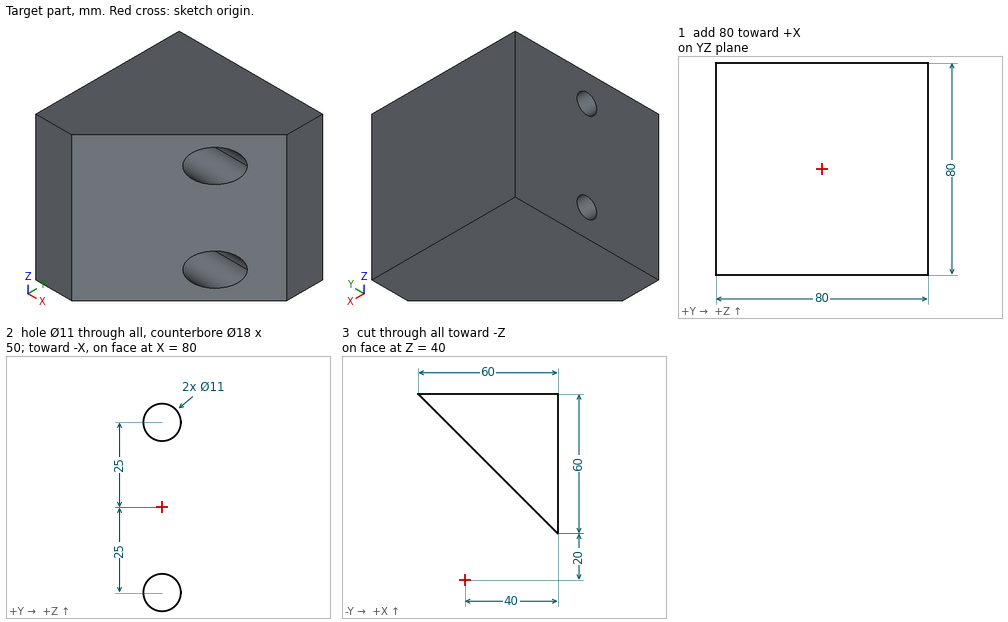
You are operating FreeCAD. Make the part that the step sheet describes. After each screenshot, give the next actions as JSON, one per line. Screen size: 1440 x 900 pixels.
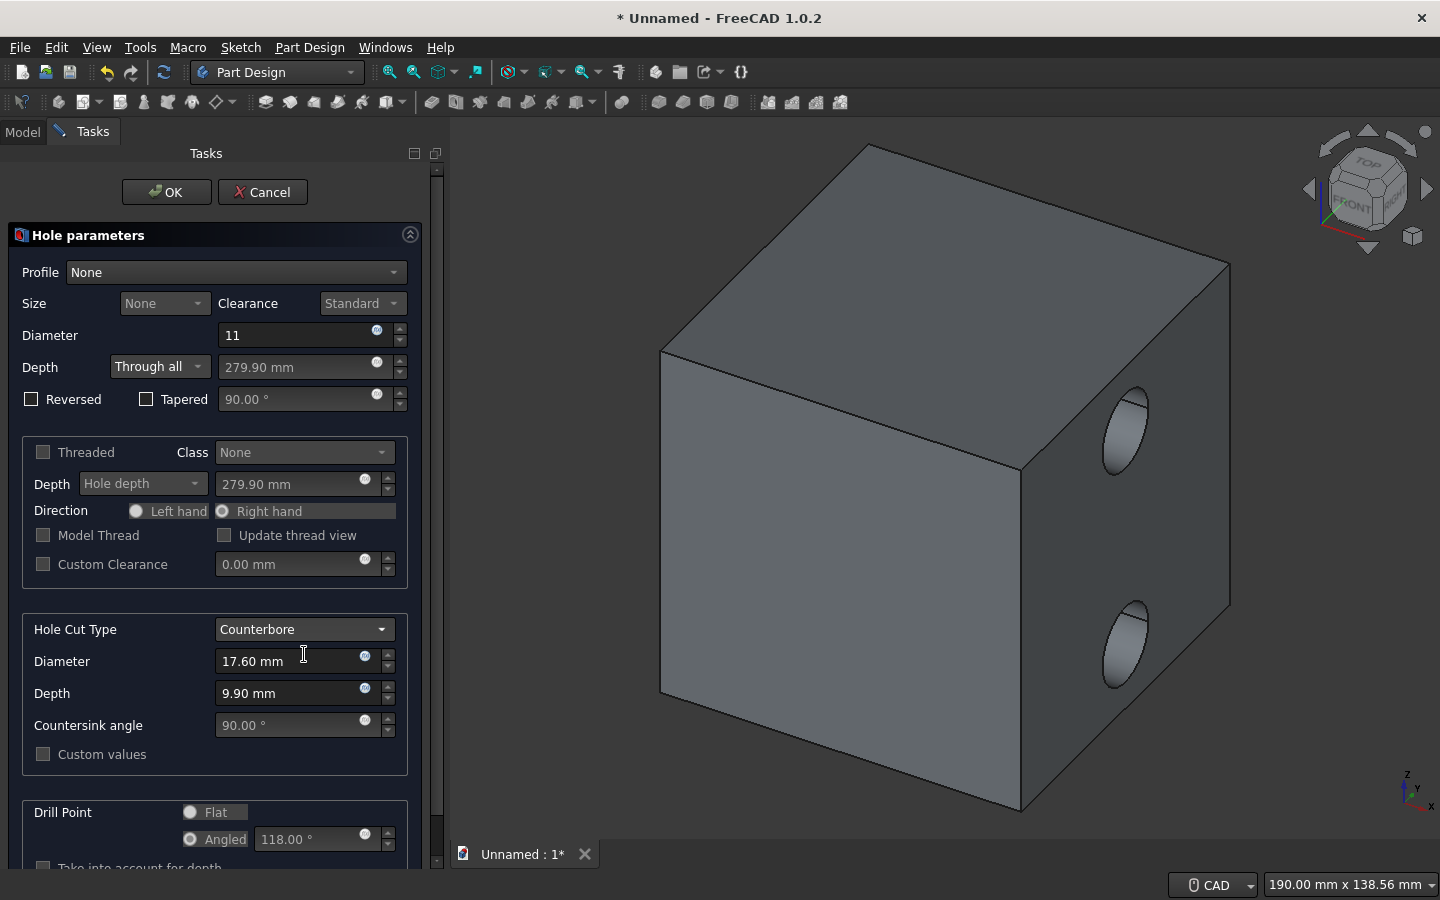
{"action": "triple_click", "coordinate": [298, 661]}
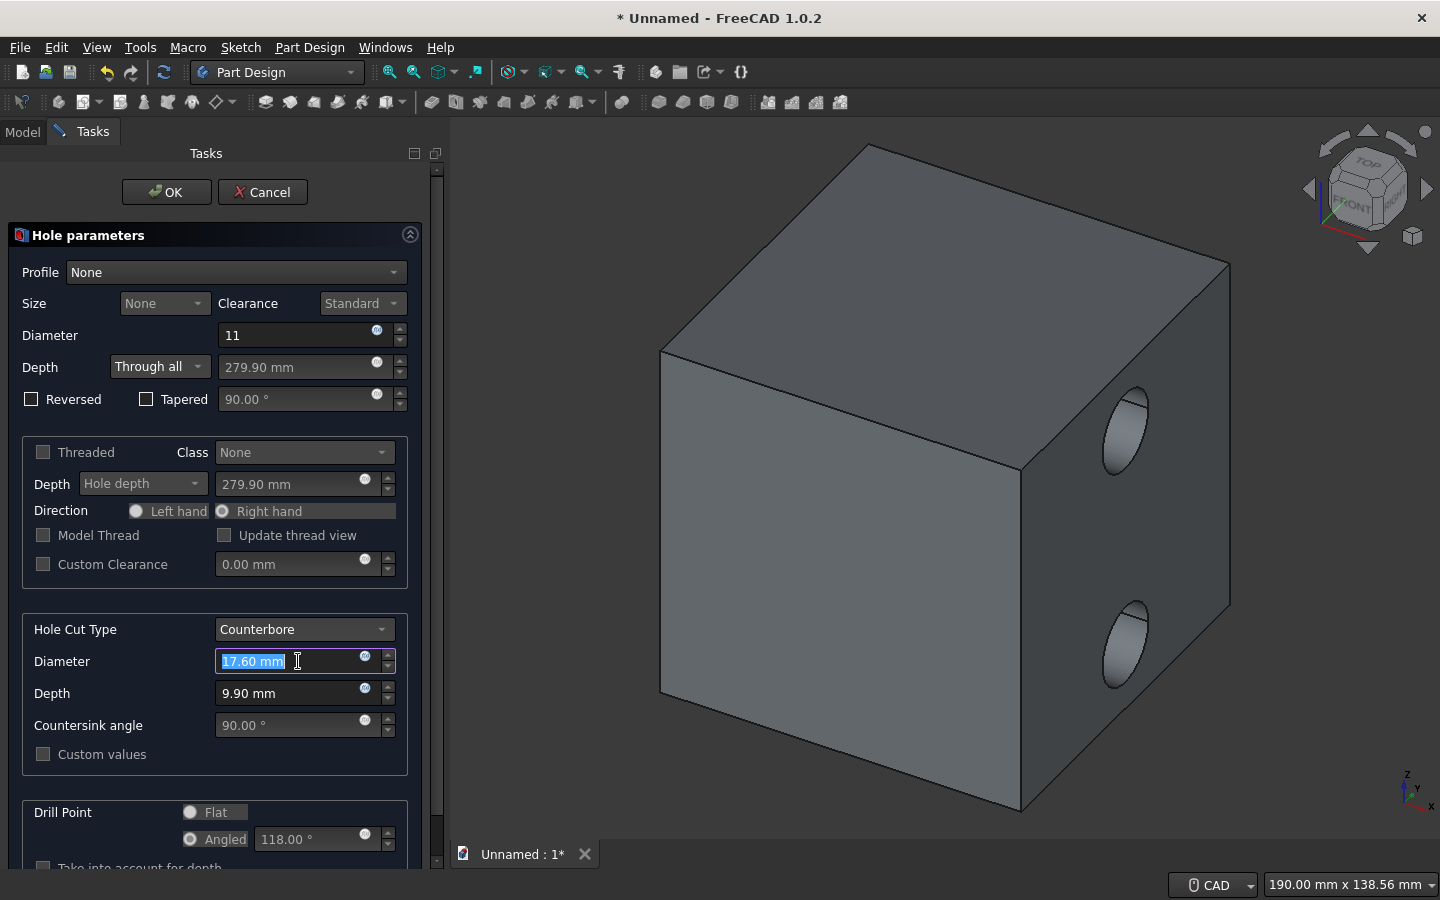
{"action": "type", "text": "18"}
{"action": "key", "text": "Tab"}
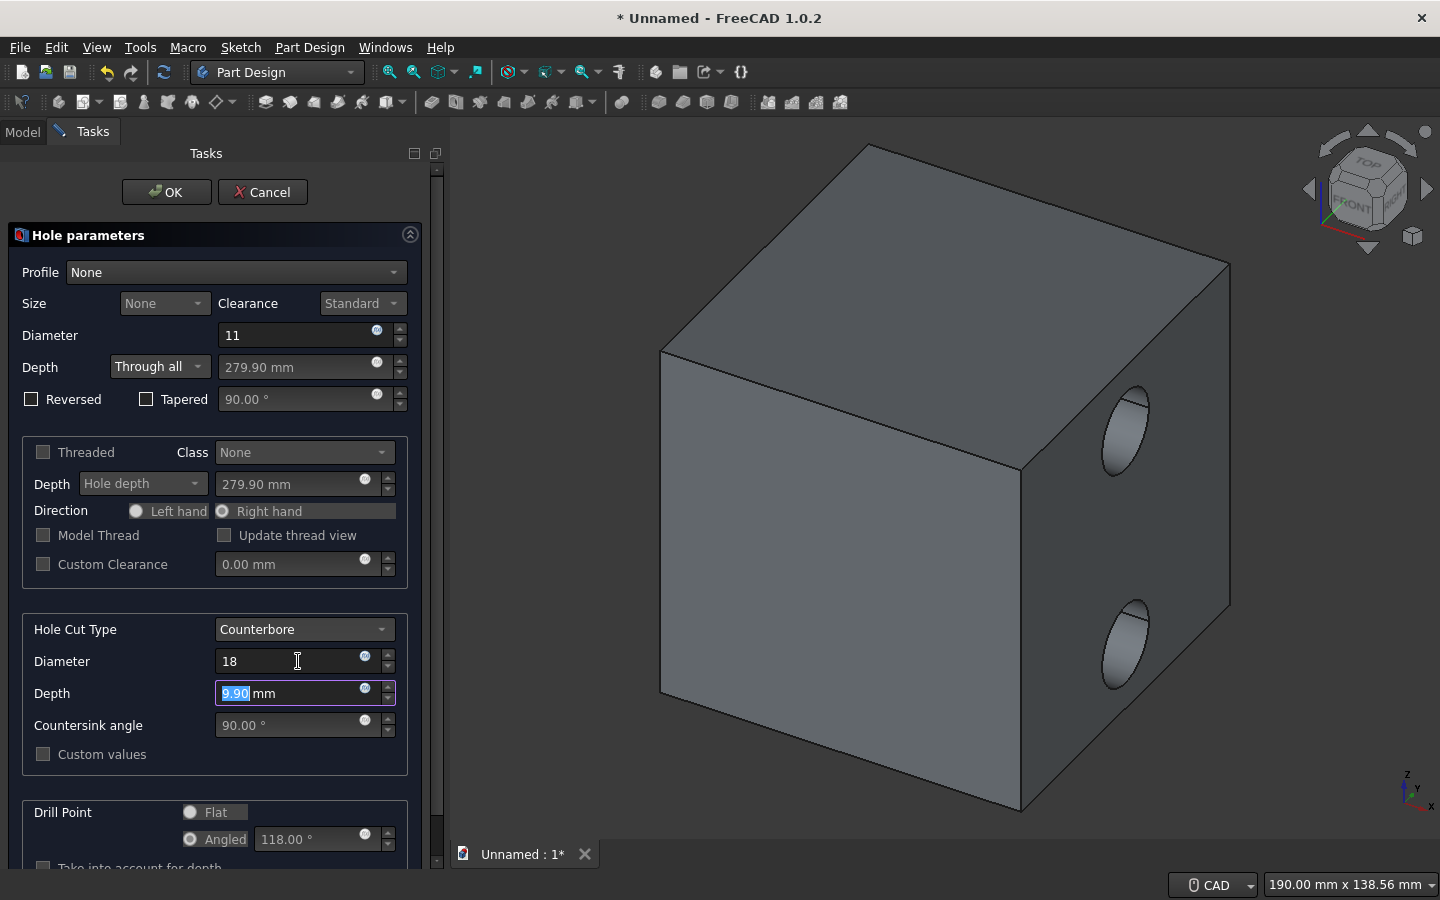
{"action": "type", "text": "50"}
{"action": "key", "text": "Tab"}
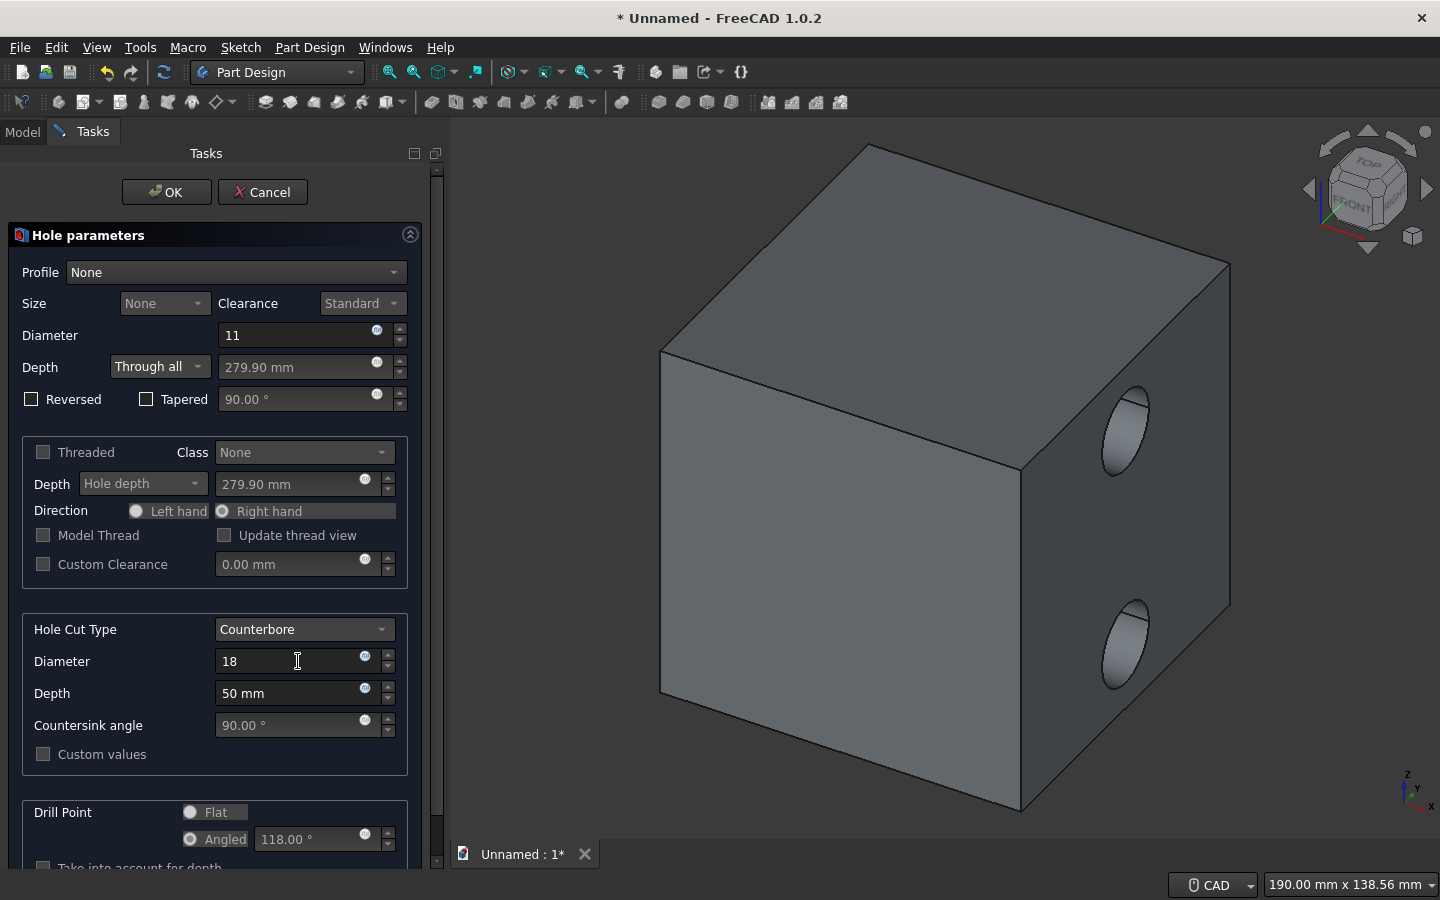
{"action": "left_click", "coordinate": [167, 192]}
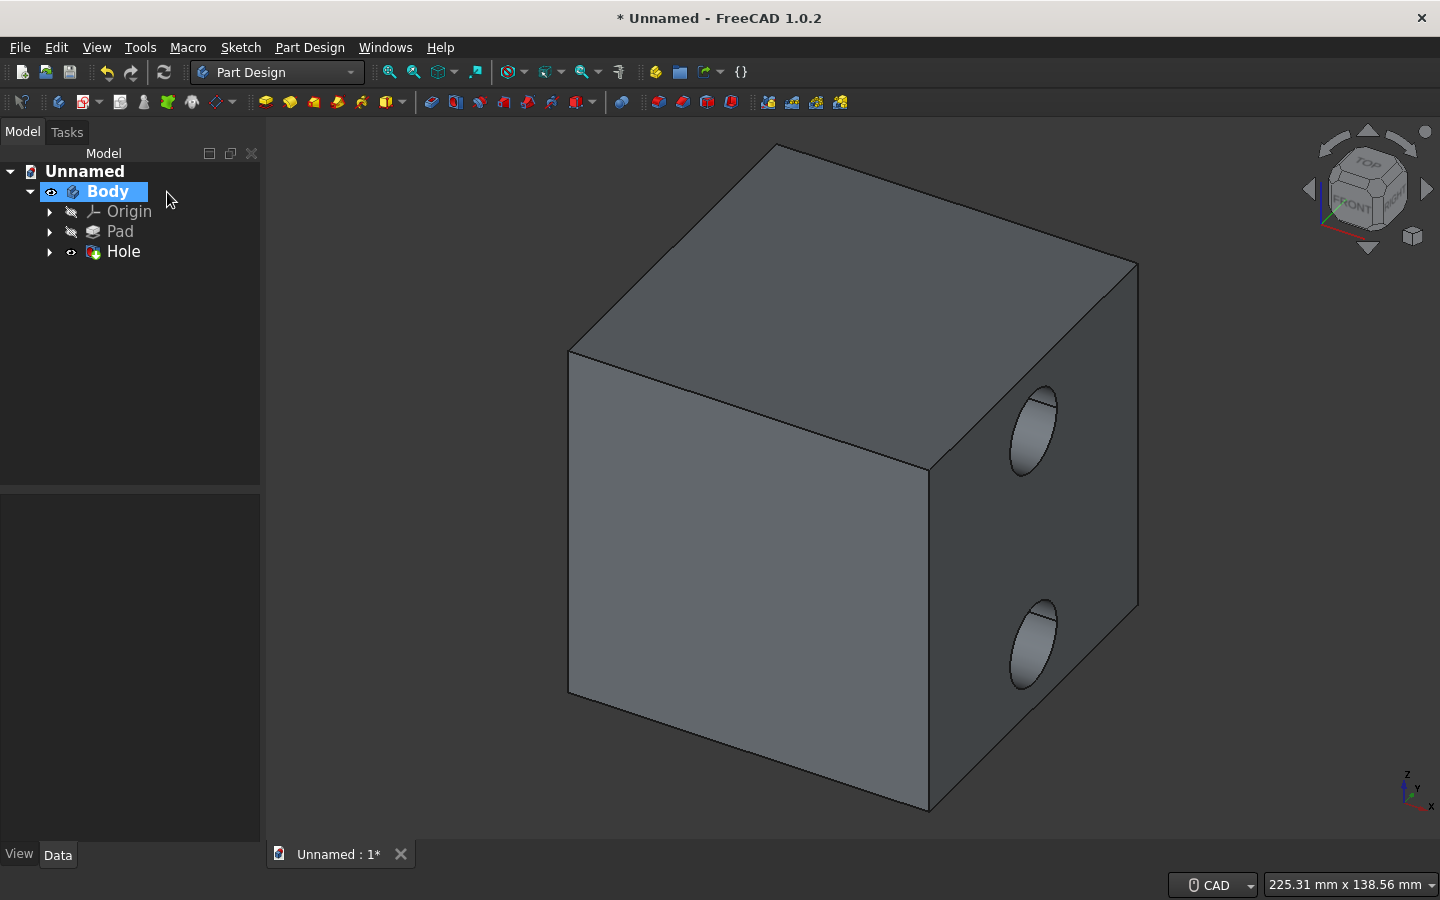
{"action": "left_click", "coordinate": [853, 306]}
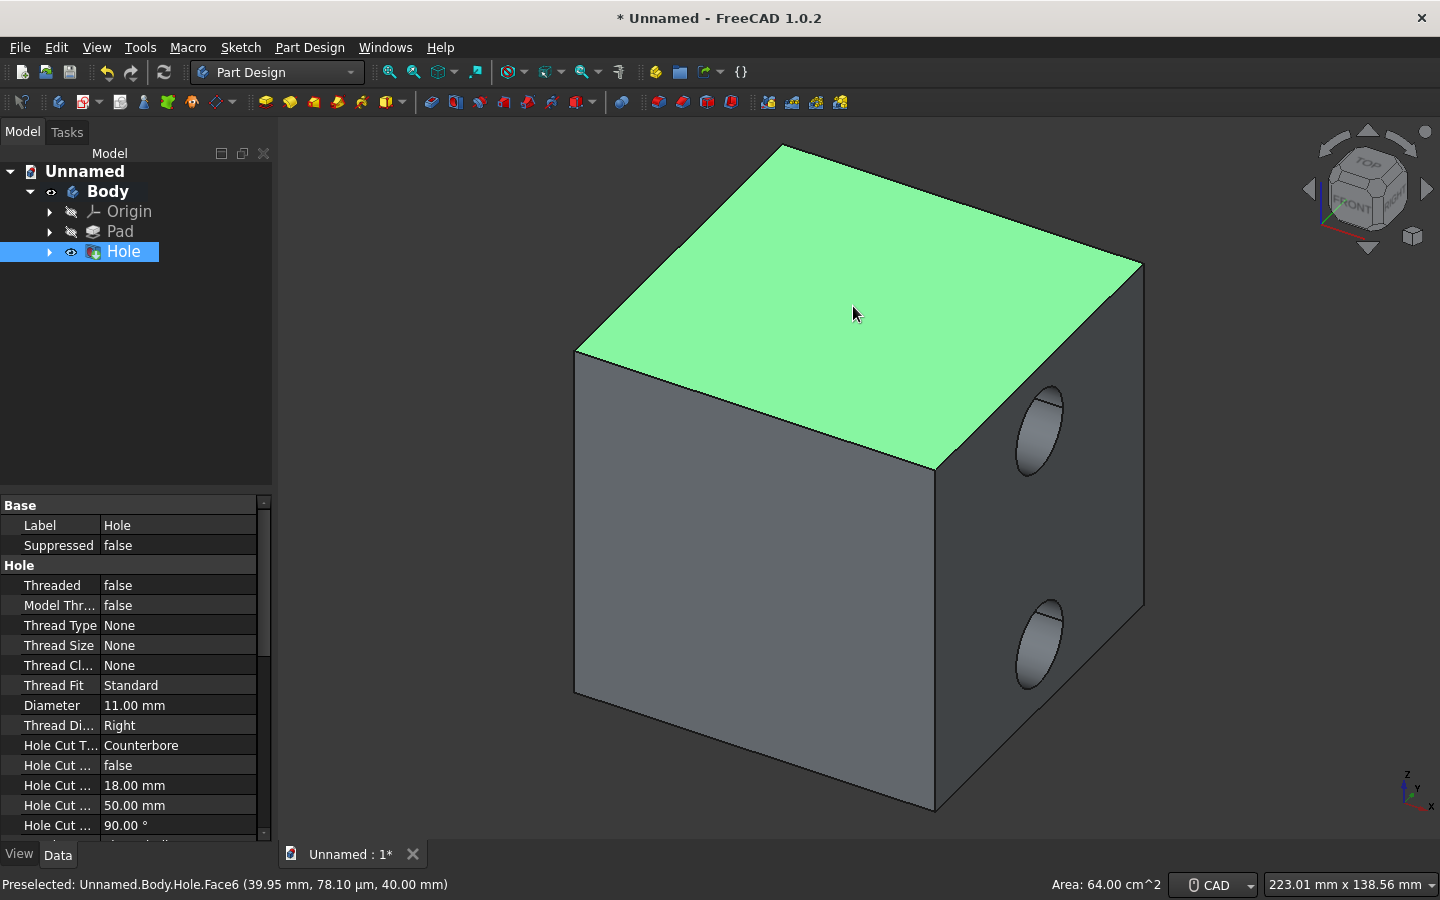
{"action": "left_click", "coordinate": [84, 102]}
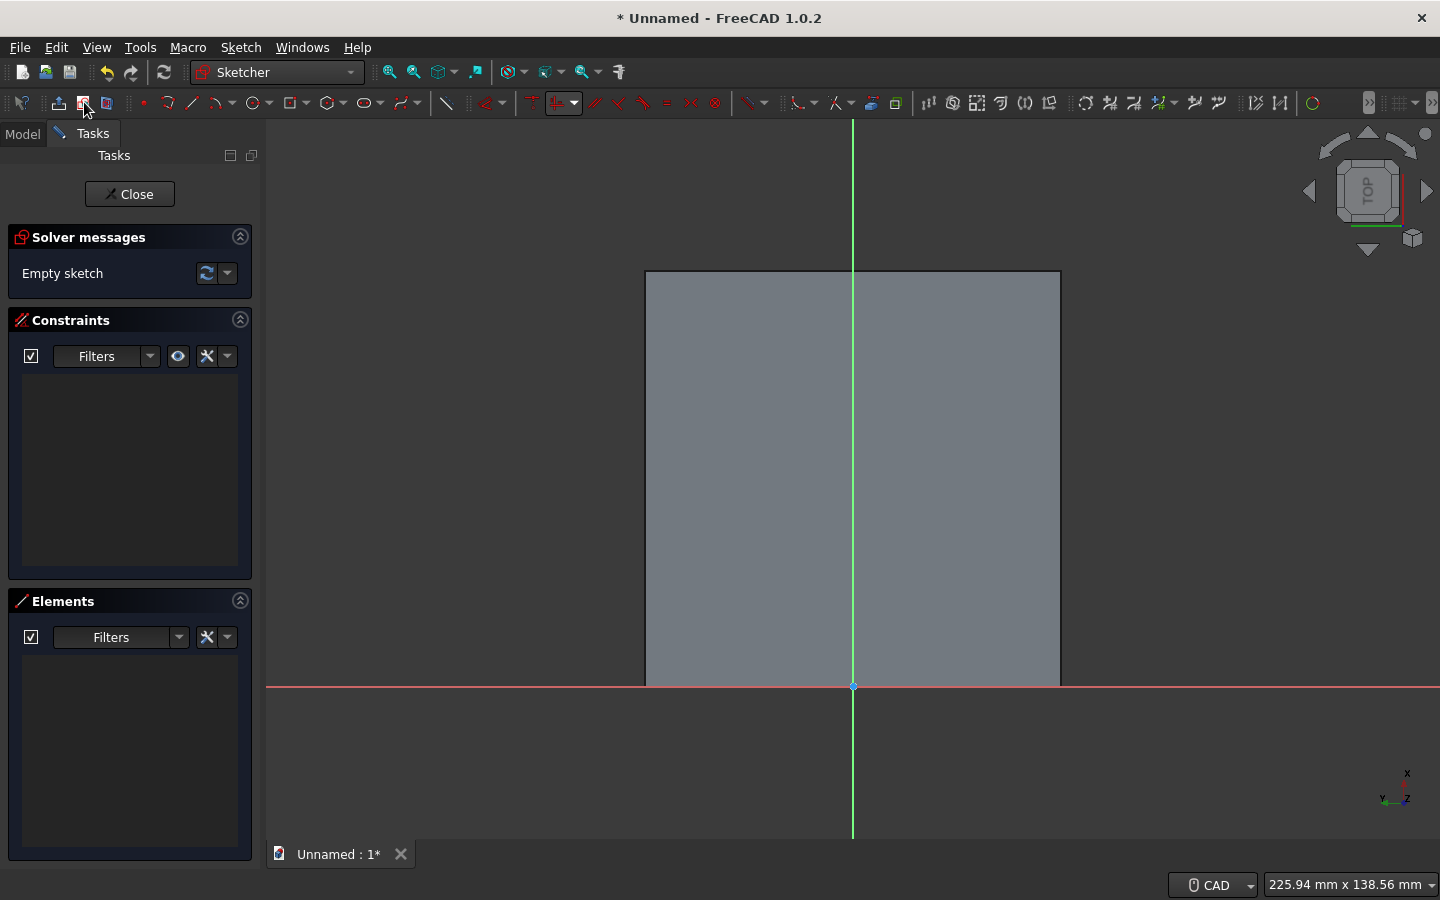
{"action": "left_click", "coordinate": [168, 104]}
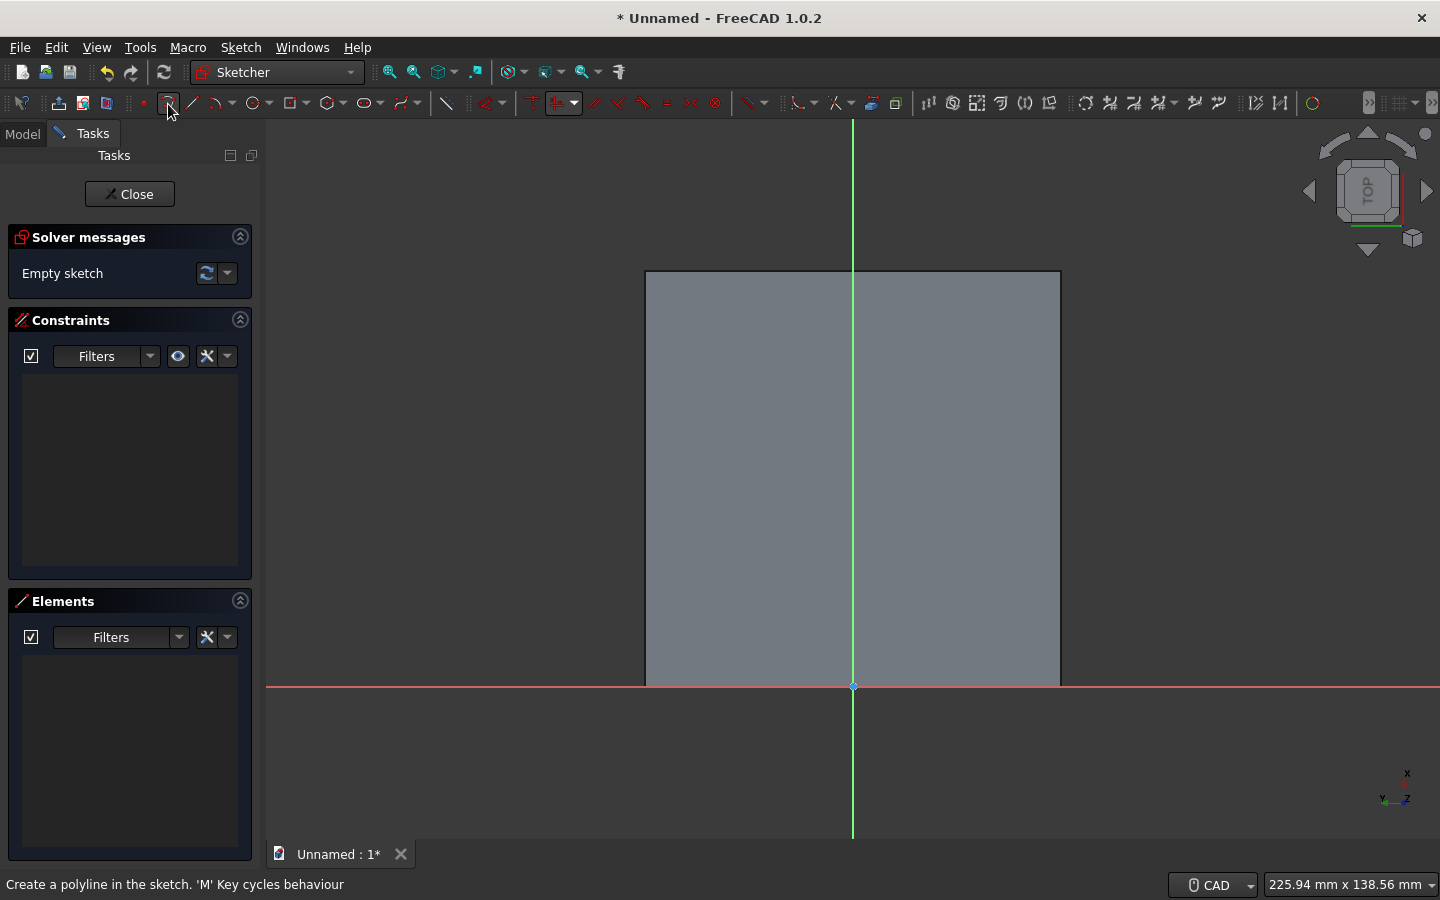
{"action": "left_click", "coordinate": [1061, 583]}
{"action": "left_click", "coordinate": [1061, 271]}
{"action": "left_click", "coordinate": [749, 271]}
{"action": "left_click", "coordinate": [1061, 584]}
{"action": "key", "text": "Escape"}
{"action": "key", "text": "Escape"}